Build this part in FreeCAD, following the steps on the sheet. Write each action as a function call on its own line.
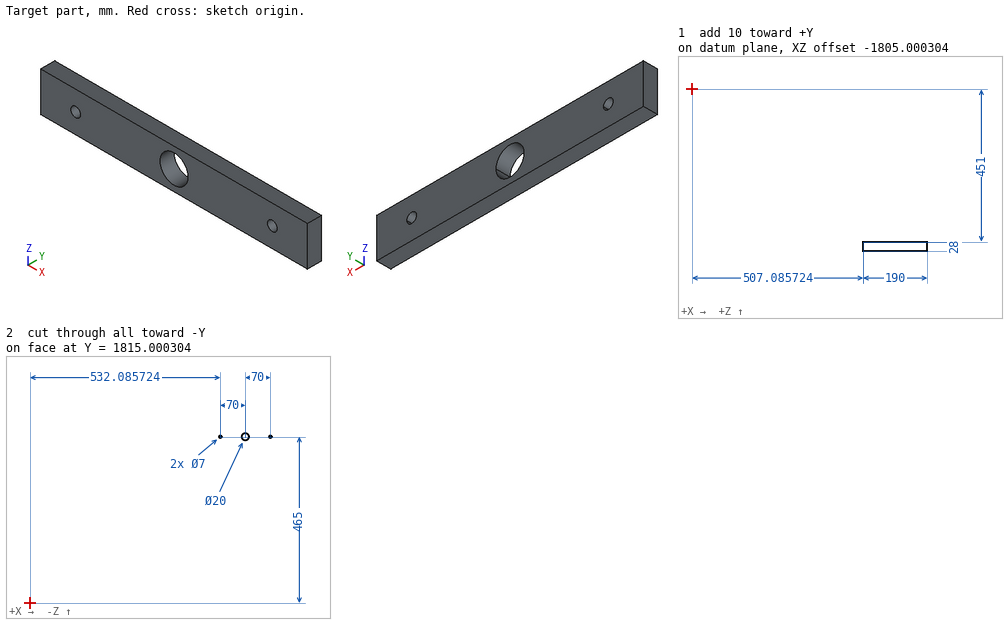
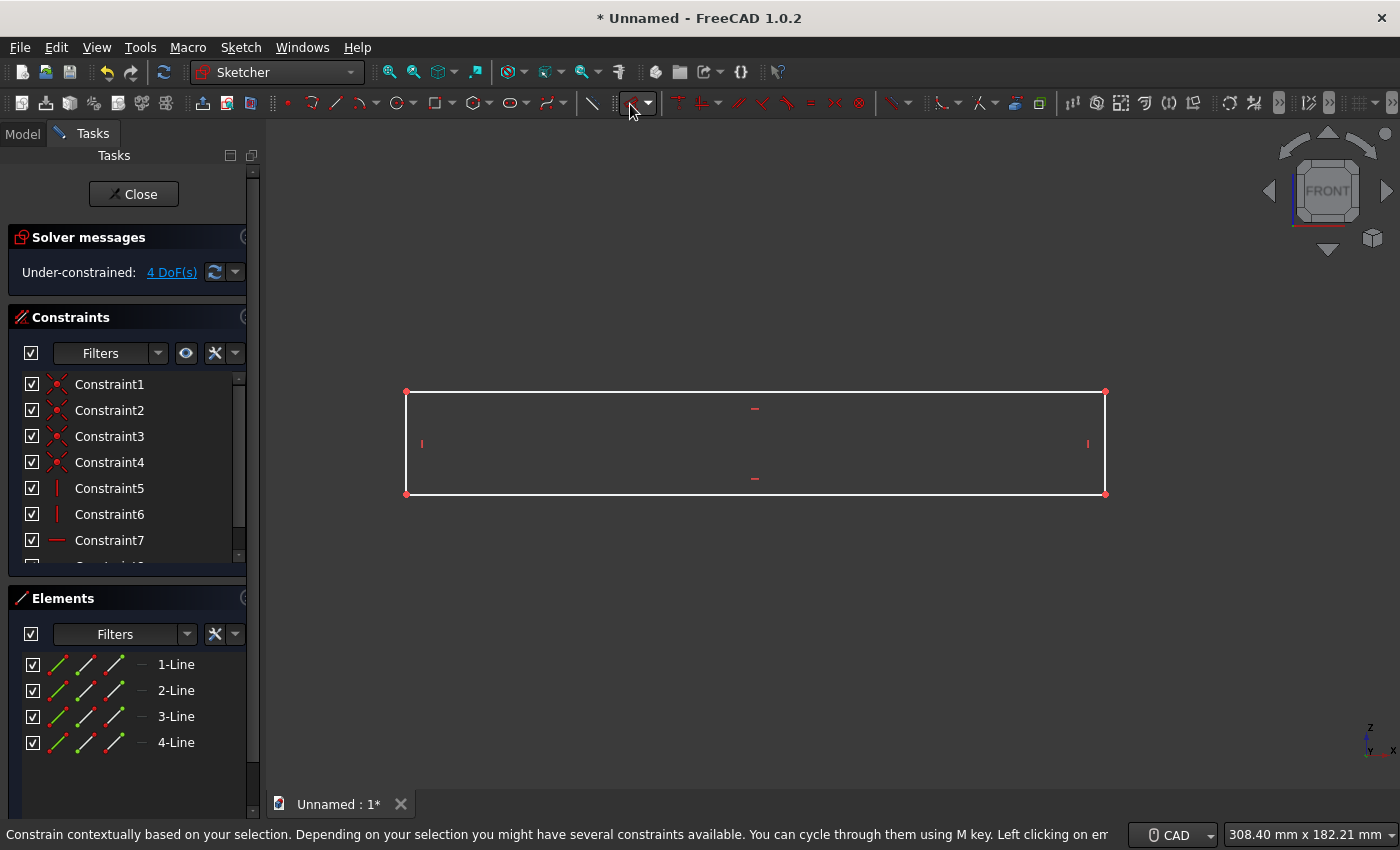
click(406, 423)
click(372, 443)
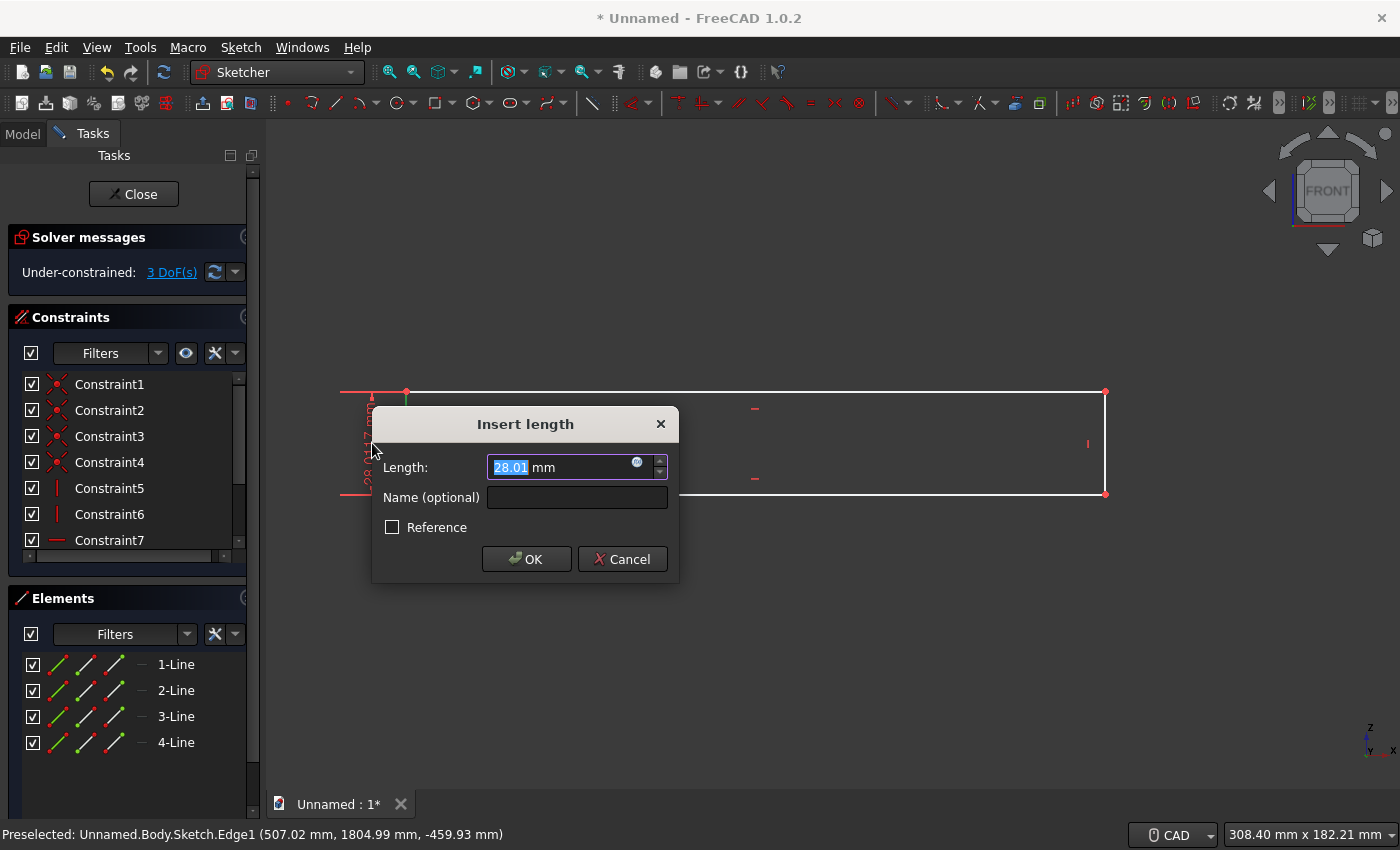
text(28)
key(Return)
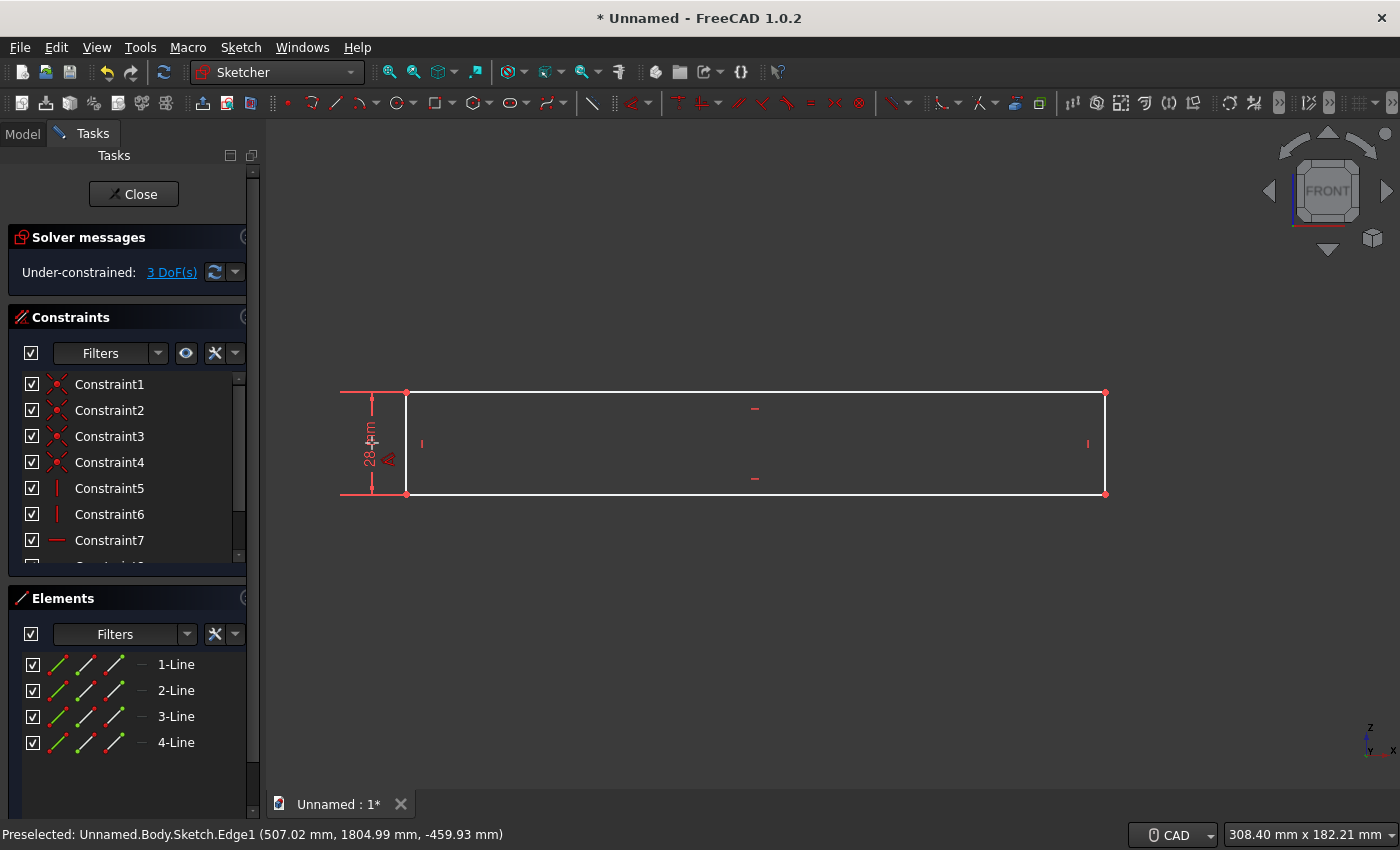
click(616, 495)
click(755, 529)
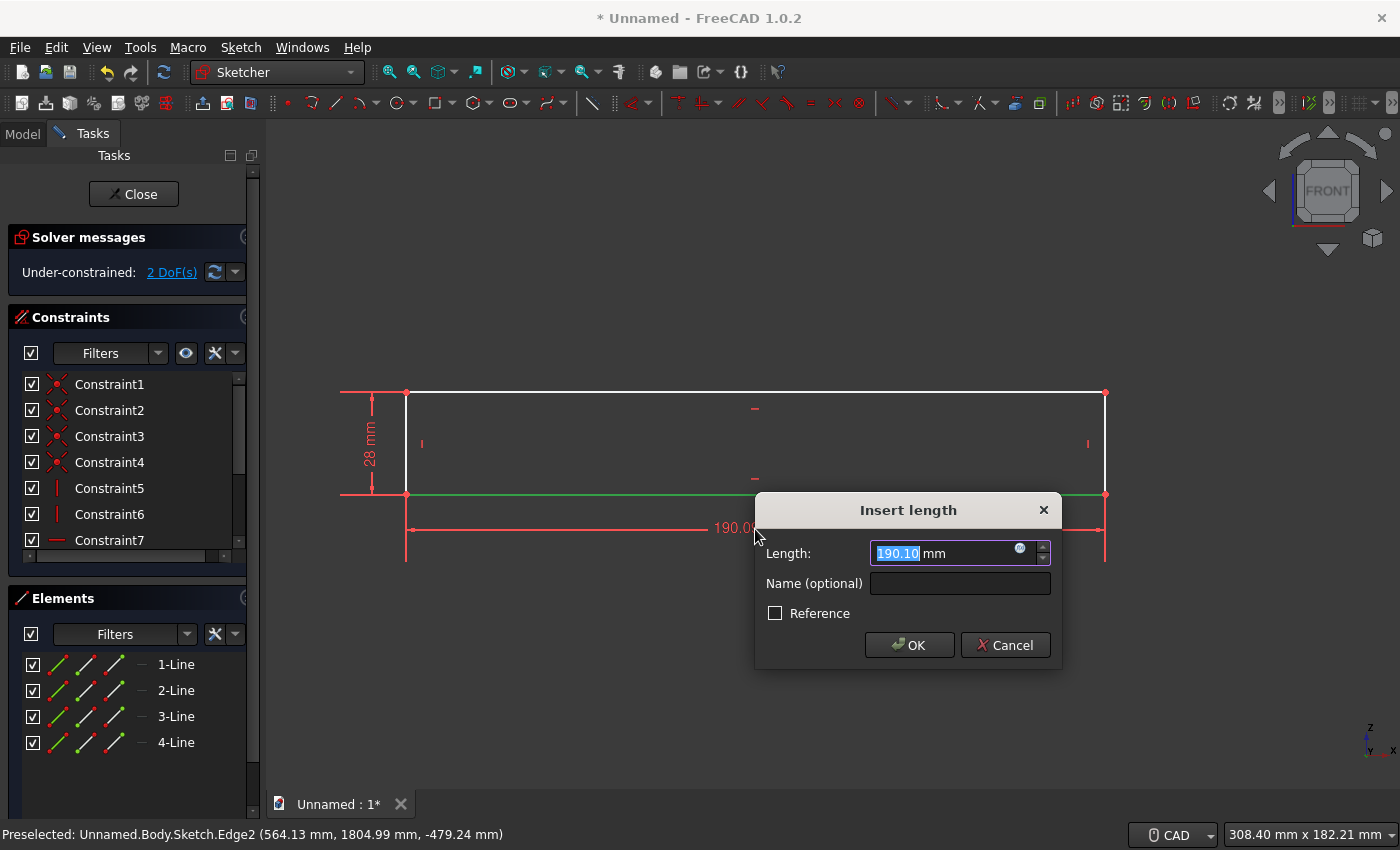
text(190)
key(Return)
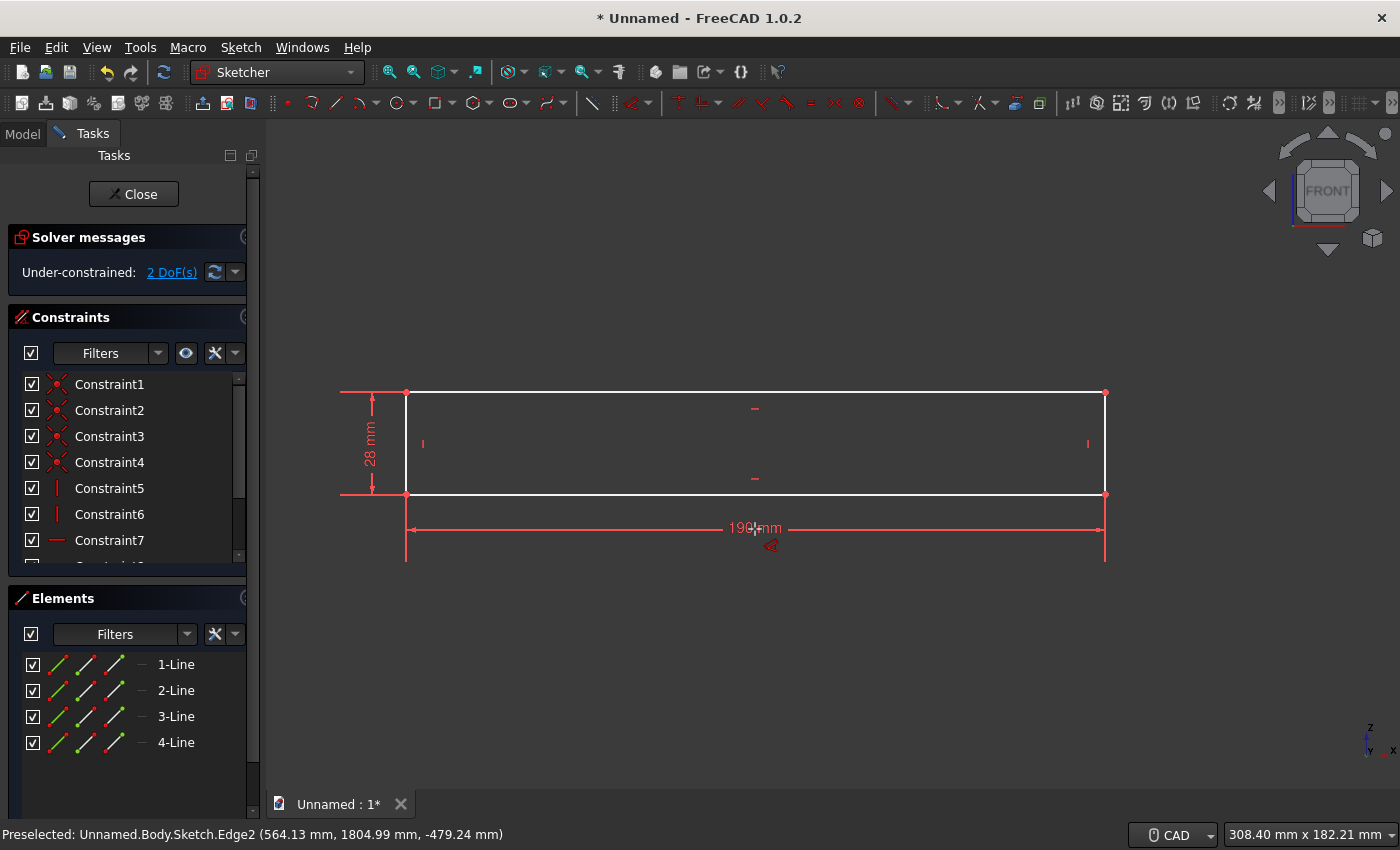
click(406, 392)
click(440, 270)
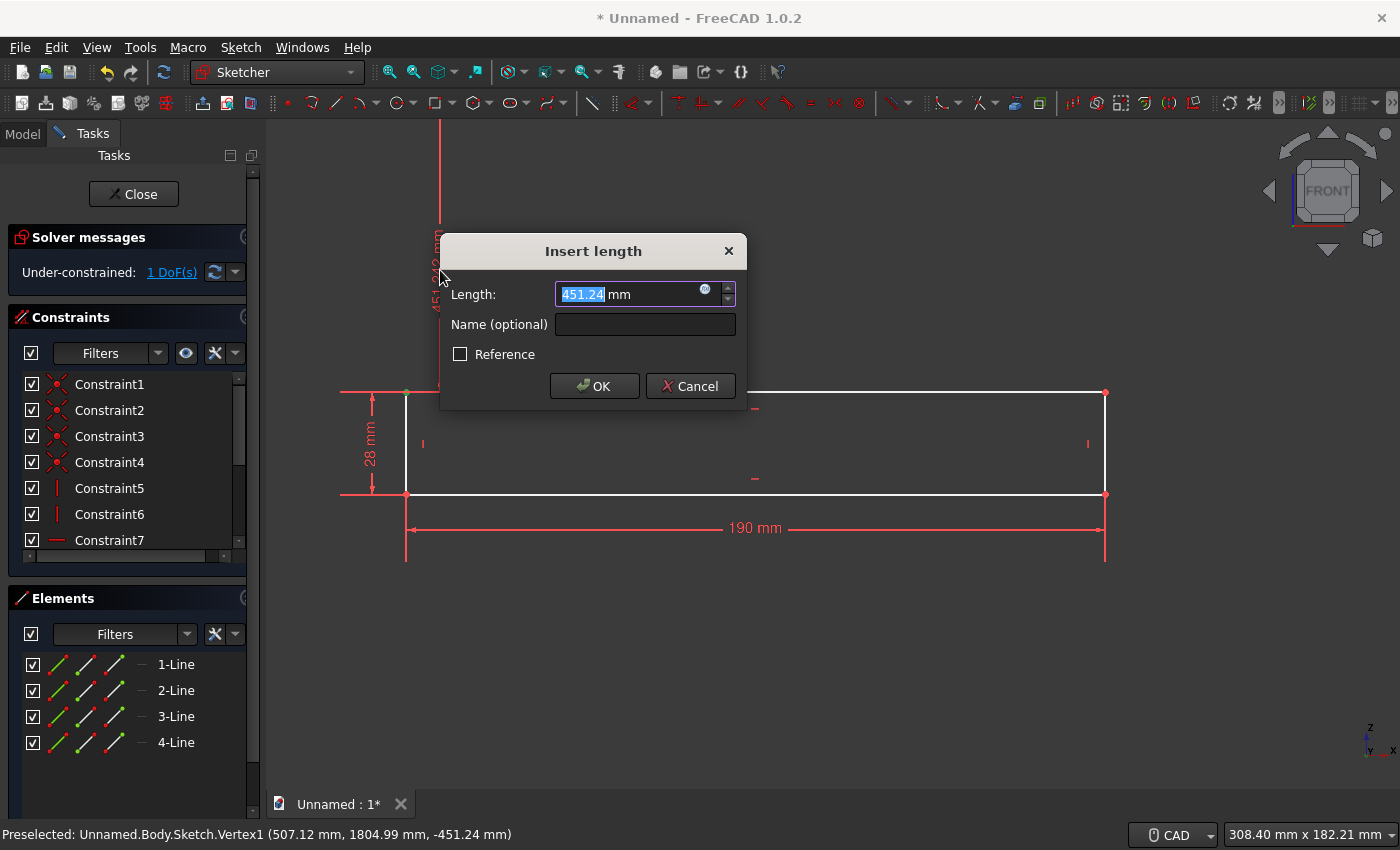
text(451)
key(Return)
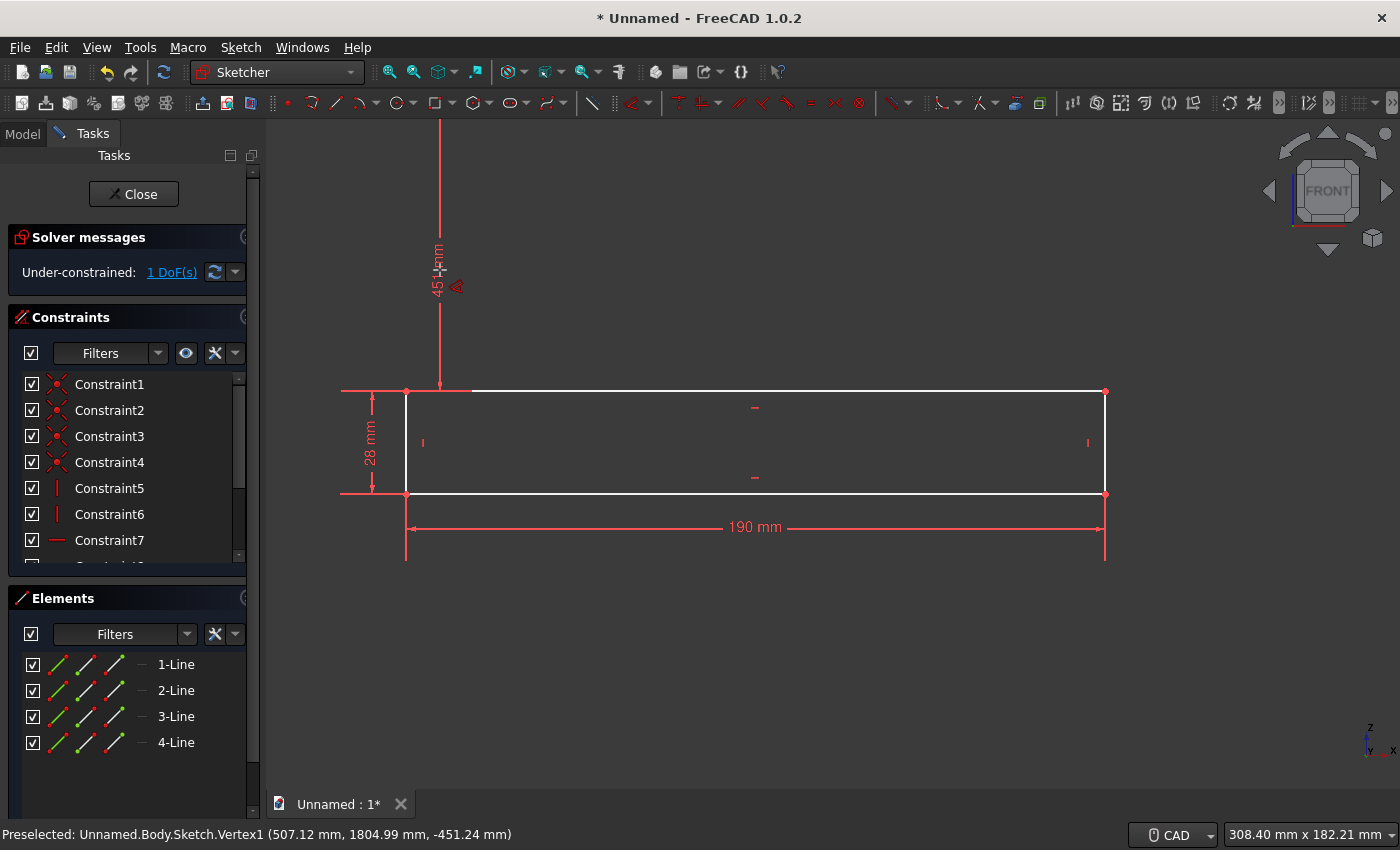
click(406, 391)
click(350, 473)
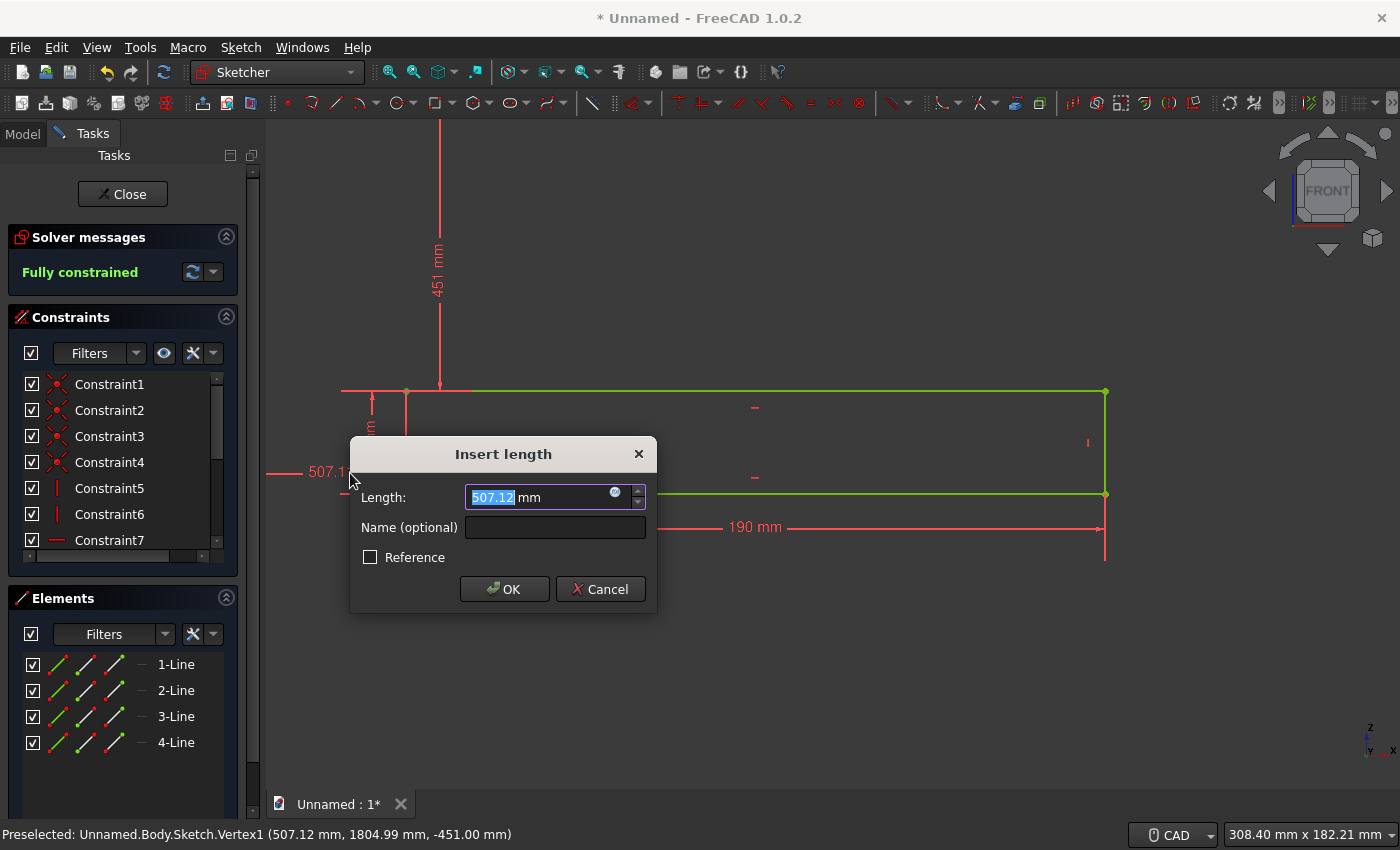
text(507.085724)
key(Return)
key(Escape)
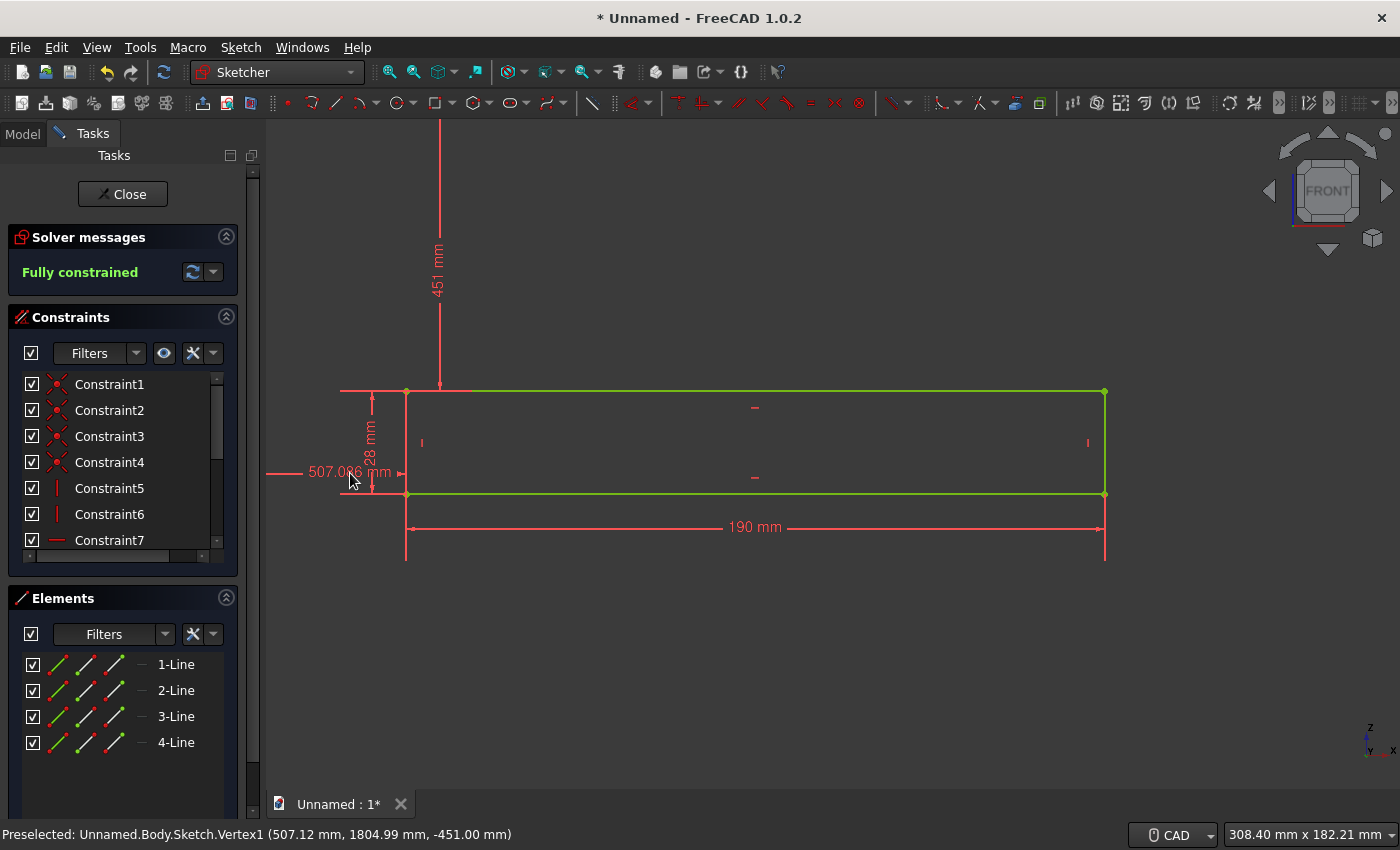
click(123, 194)